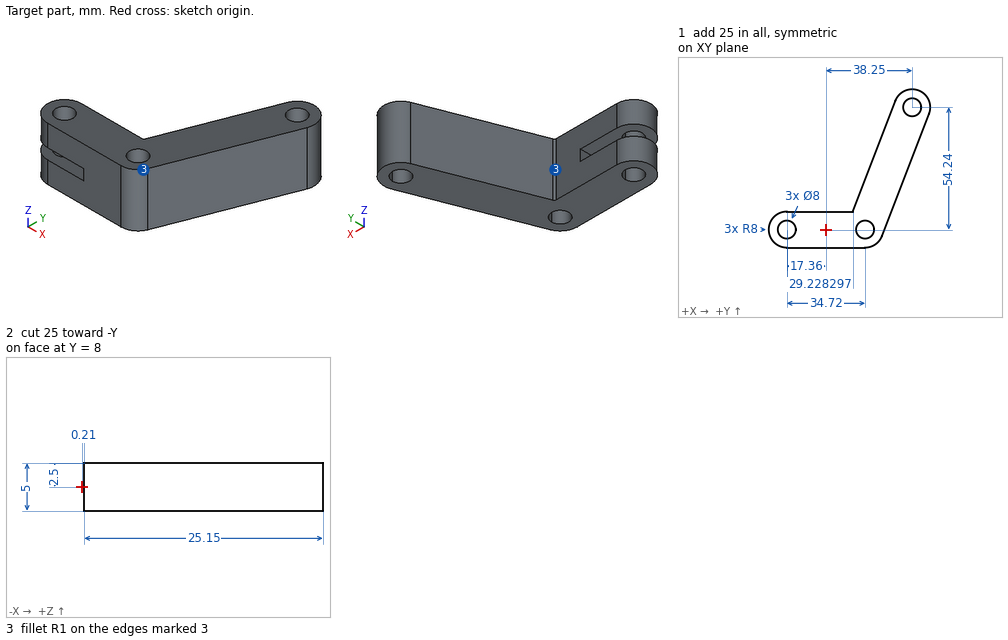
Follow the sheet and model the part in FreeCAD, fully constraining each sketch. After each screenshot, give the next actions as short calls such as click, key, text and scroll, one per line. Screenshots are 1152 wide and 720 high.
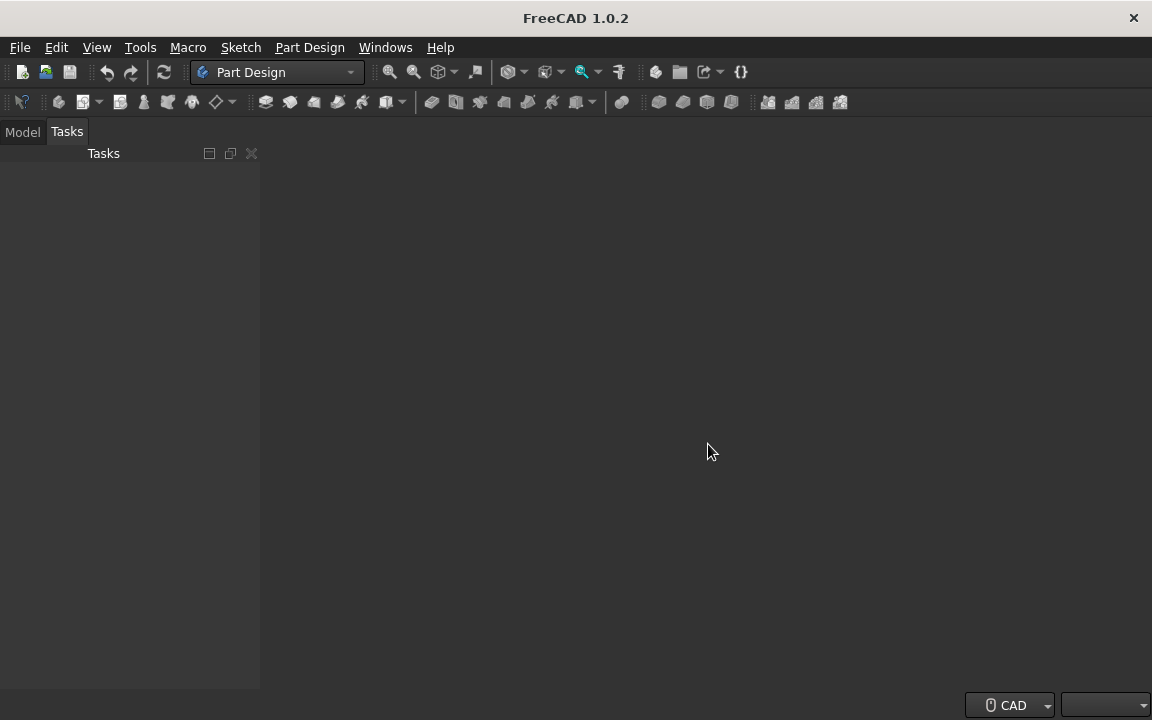
click(22, 72)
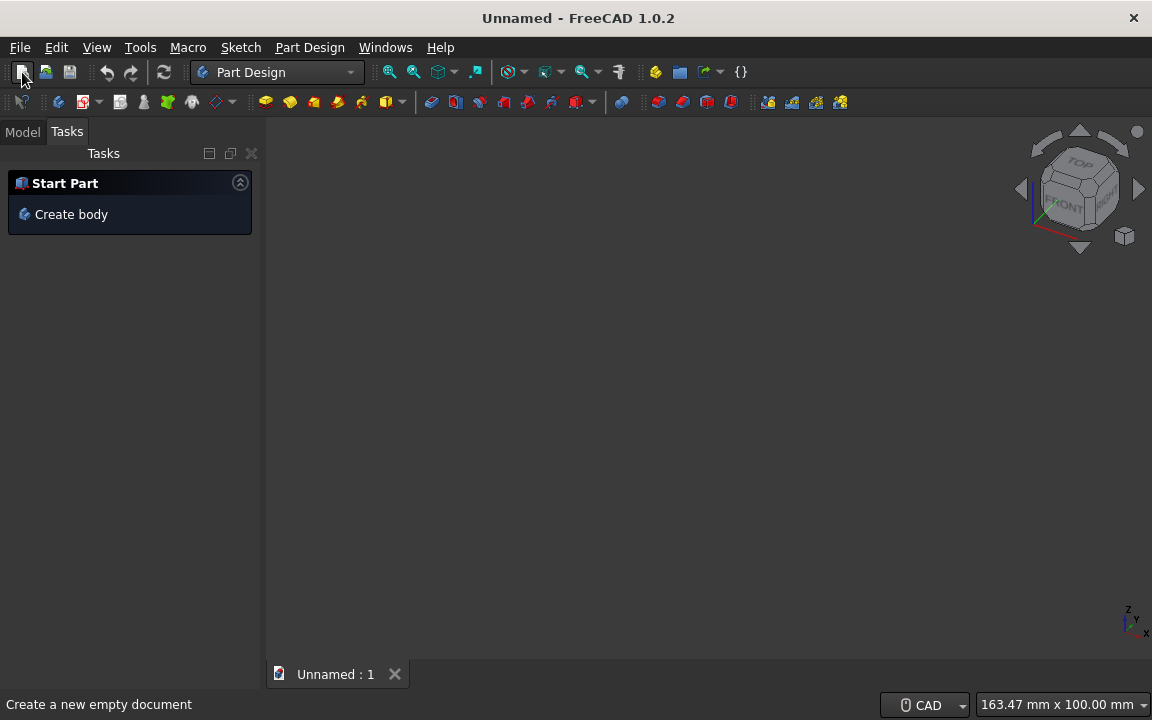
click(84, 102)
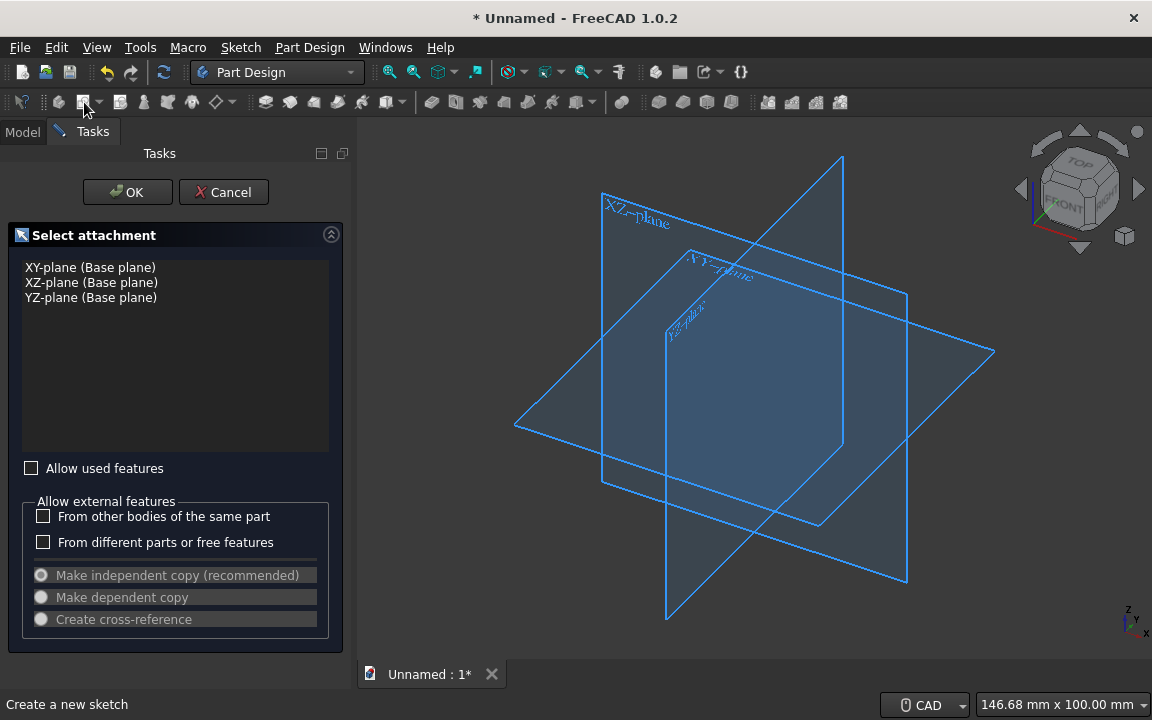
click(82, 268)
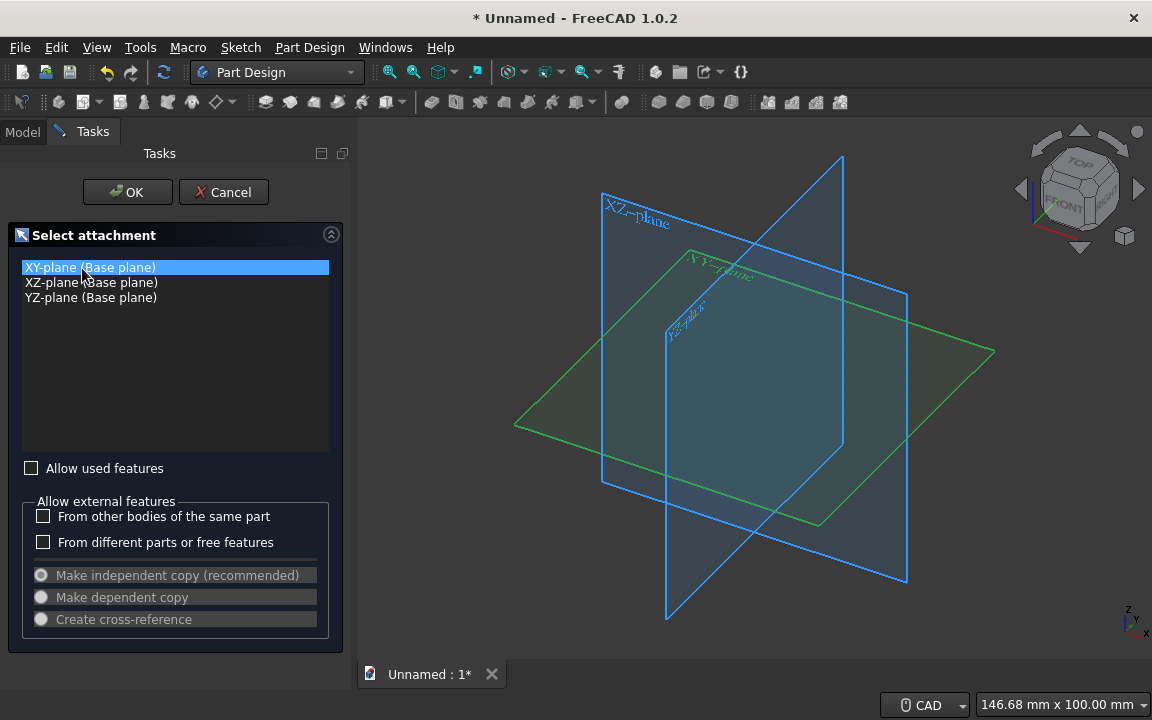
click(128, 192)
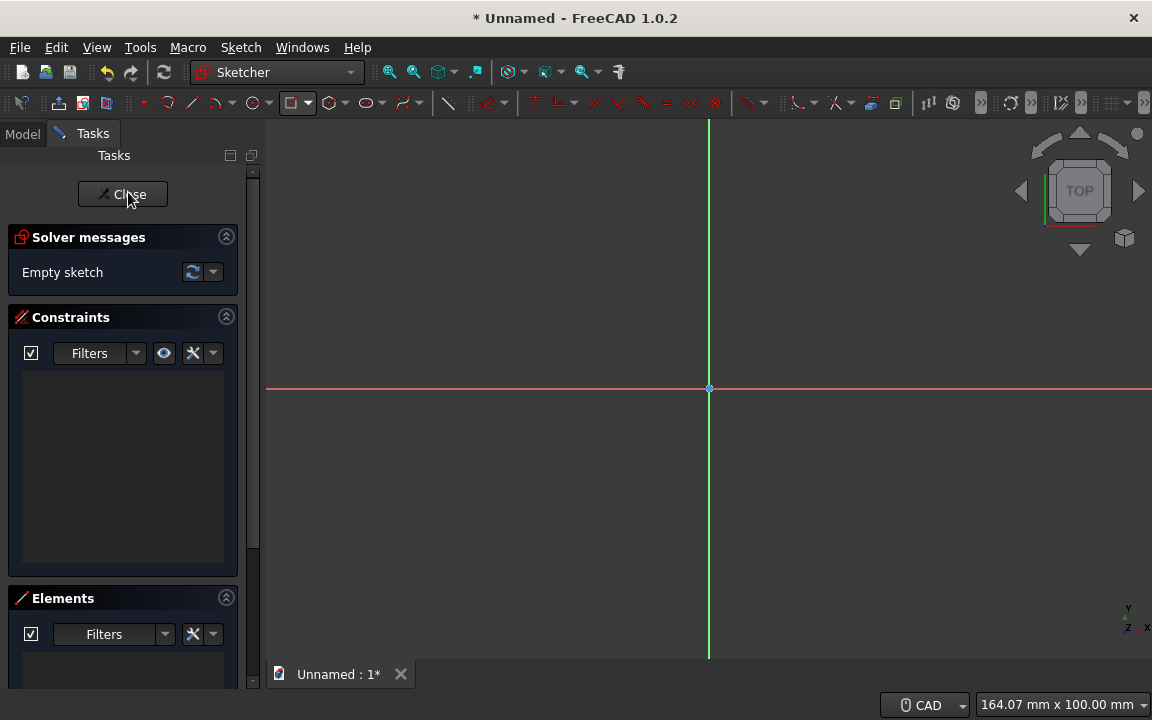
scroll(389, 631, down, 2)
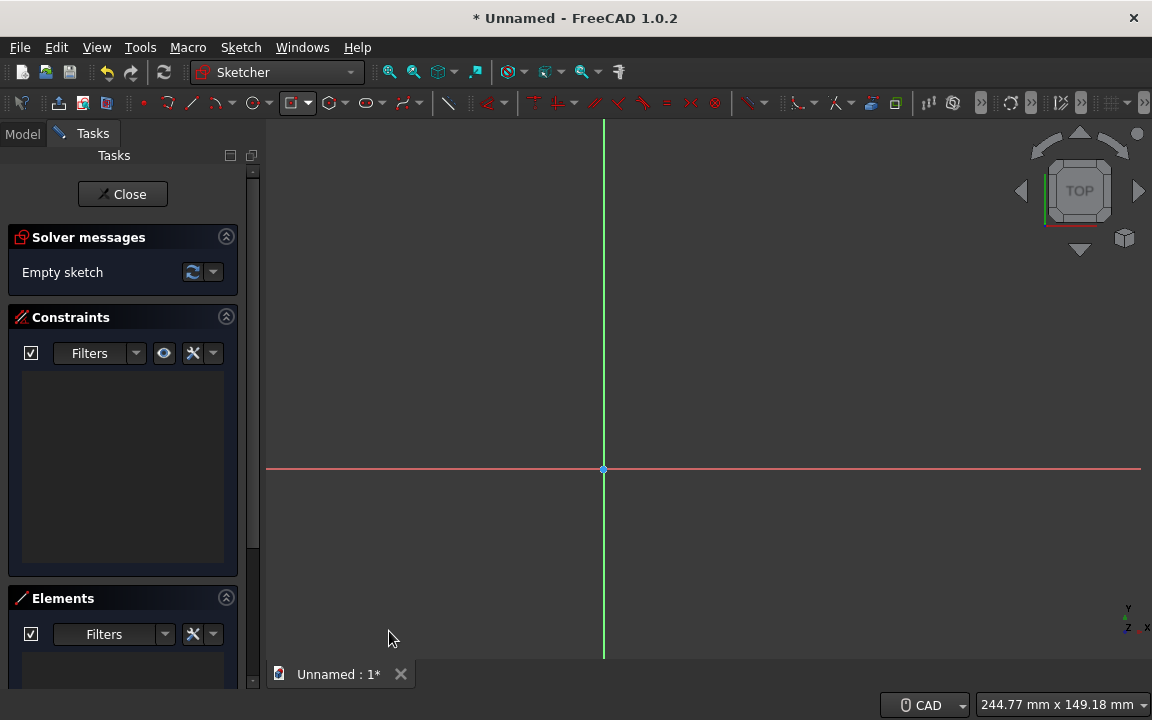
scroll(640, 337, up, 2)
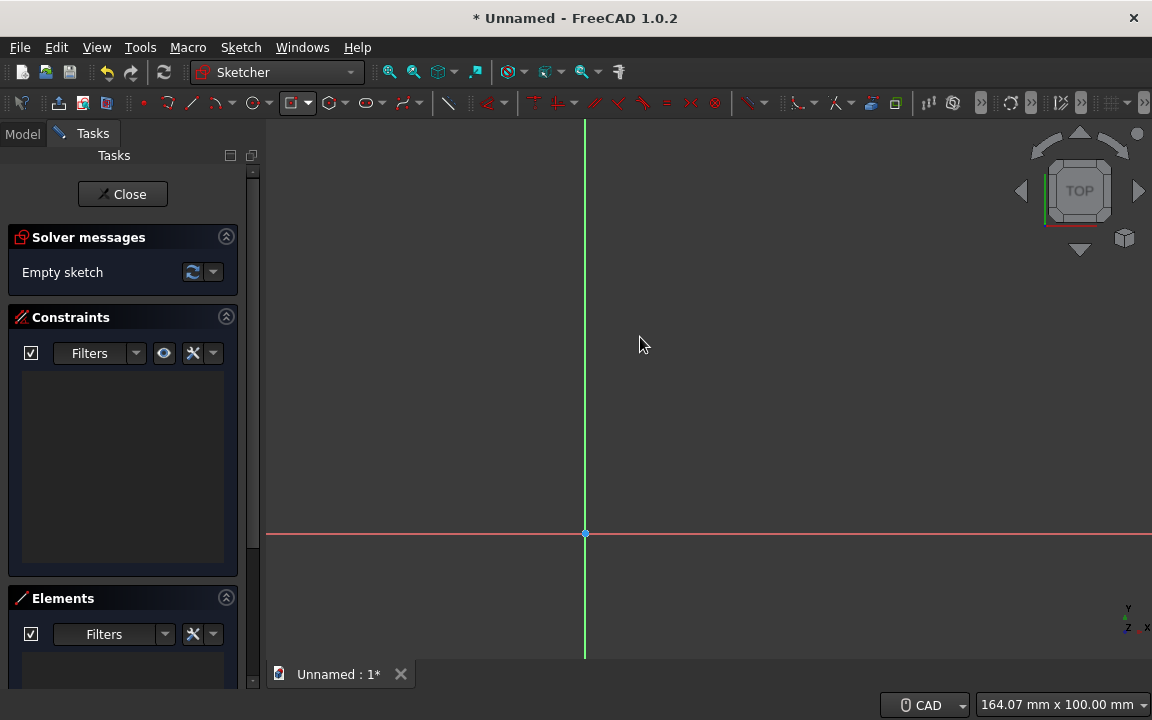
click(192, 104)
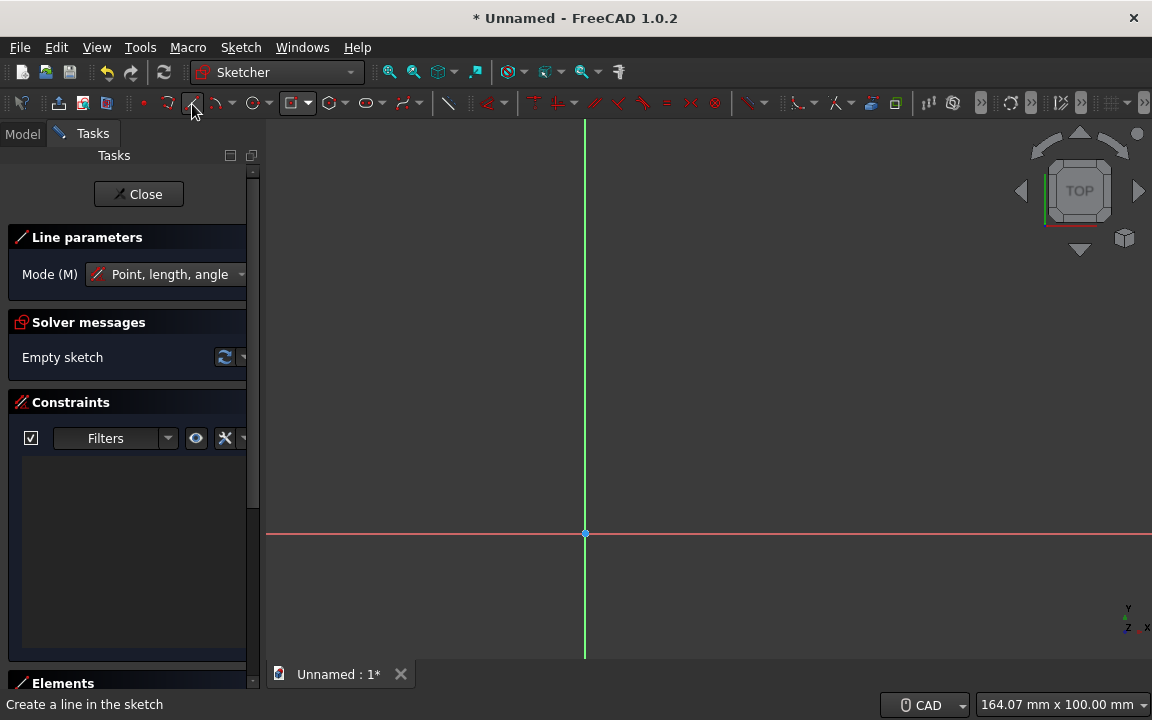
click(719, 549)
click(832, 256)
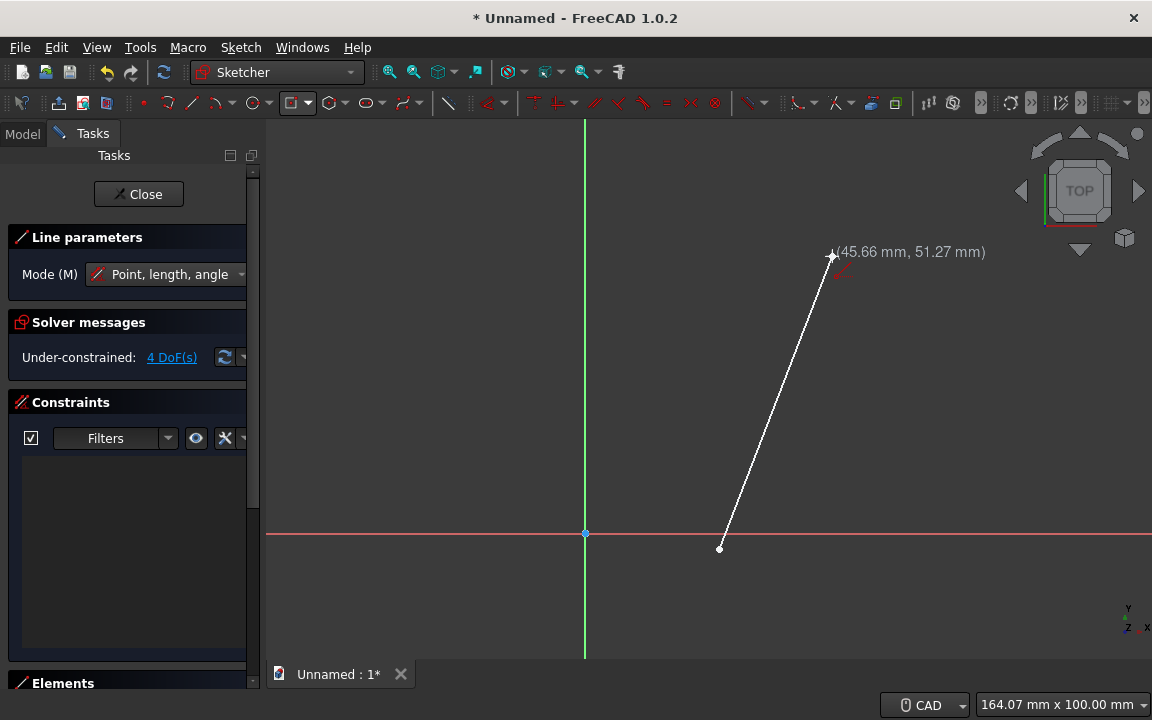
click(168, 104)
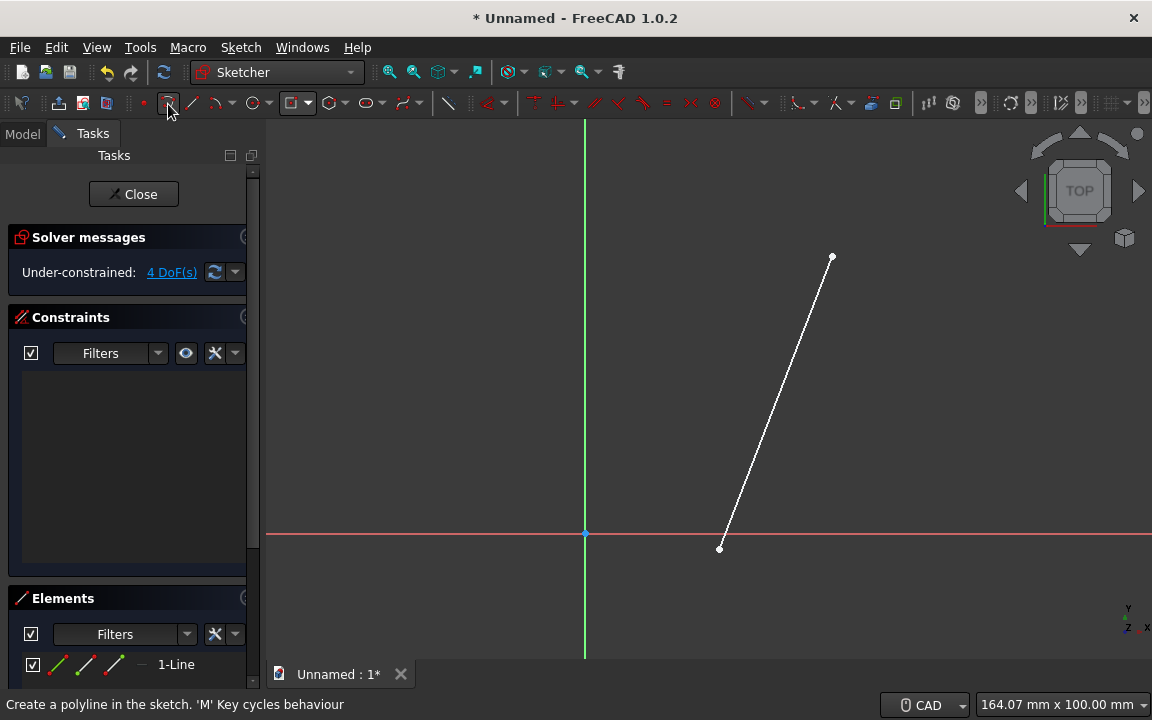
click(752, 225)
click(650, 491)
click(492, 491)
right_click(492, 491)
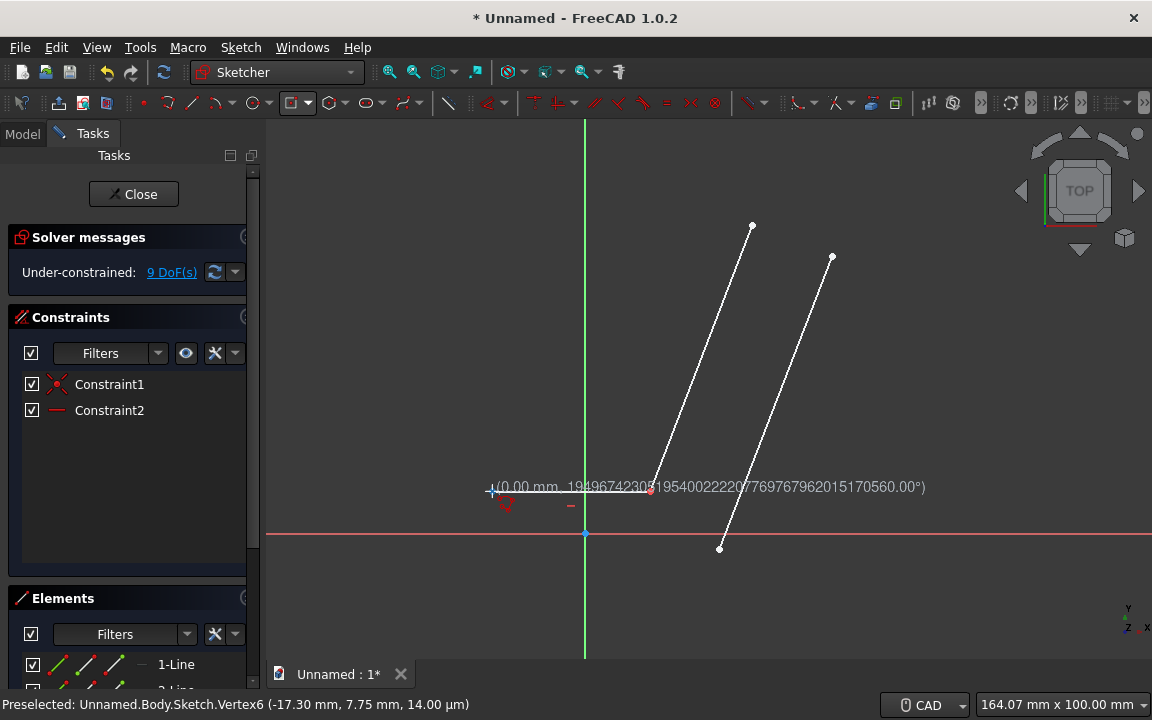
click(192, 104)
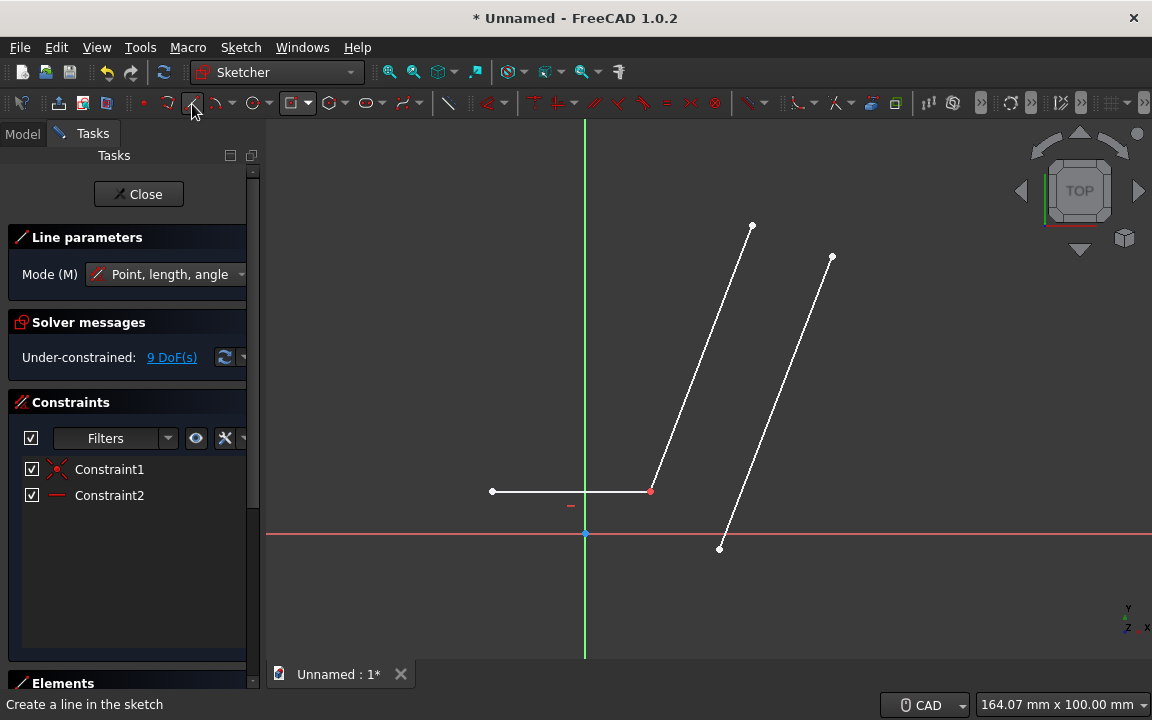
click(492, 577)
click(679, 577)